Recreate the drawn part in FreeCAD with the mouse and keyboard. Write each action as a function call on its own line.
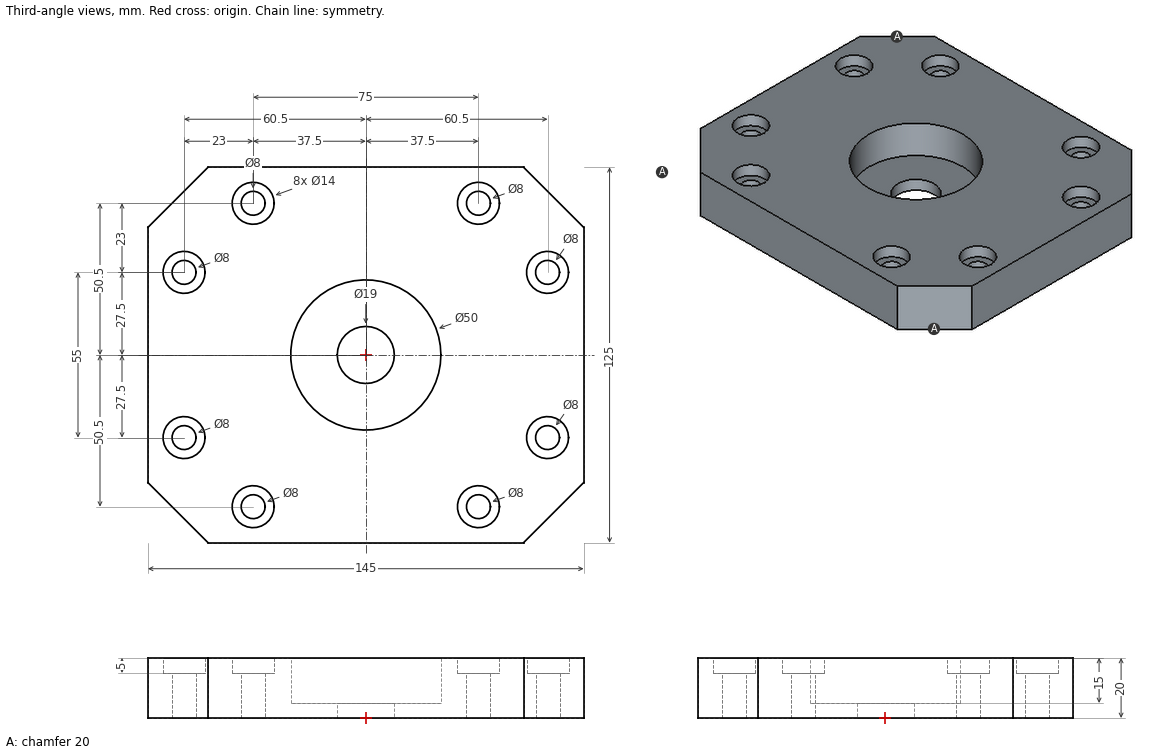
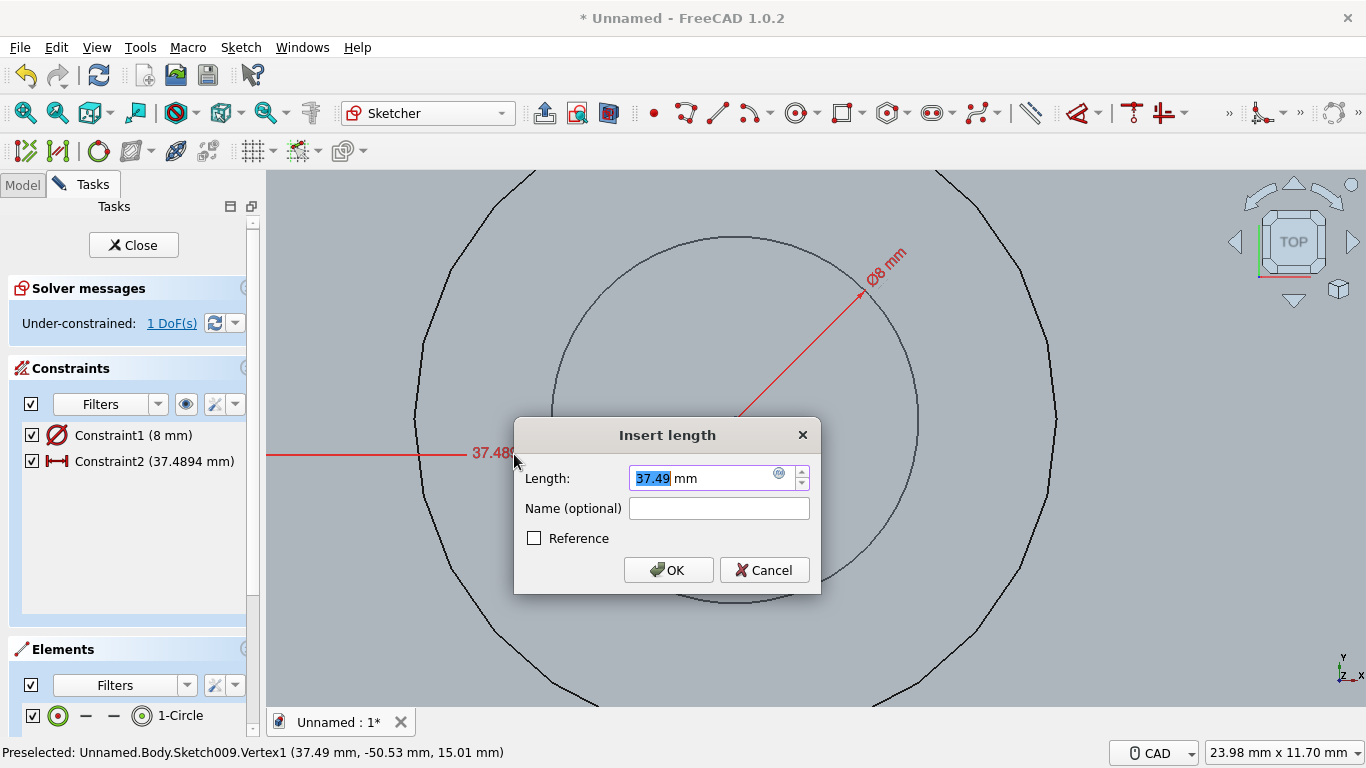
text(37.5)
key(Return)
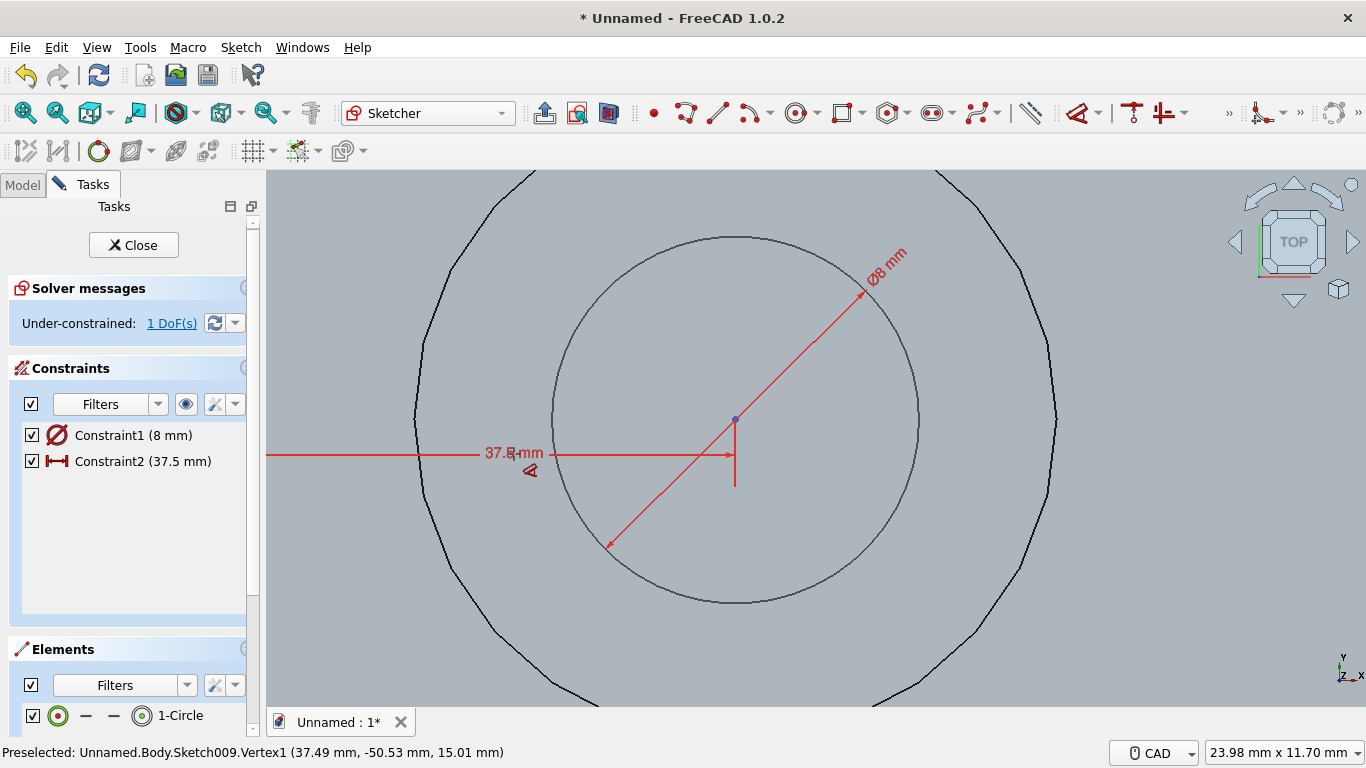
click(735, 420)
click(769, 309)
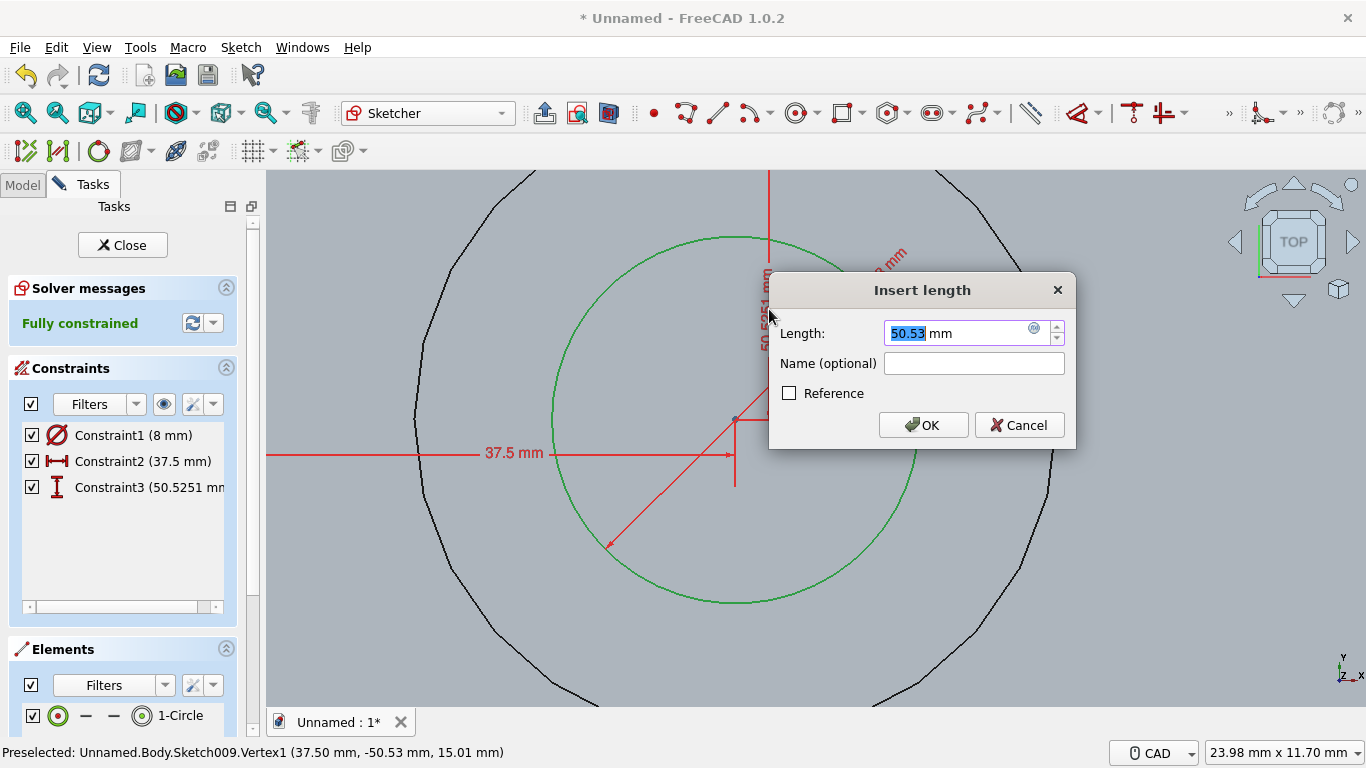
text(50.5)
key(Return)
key(Escape)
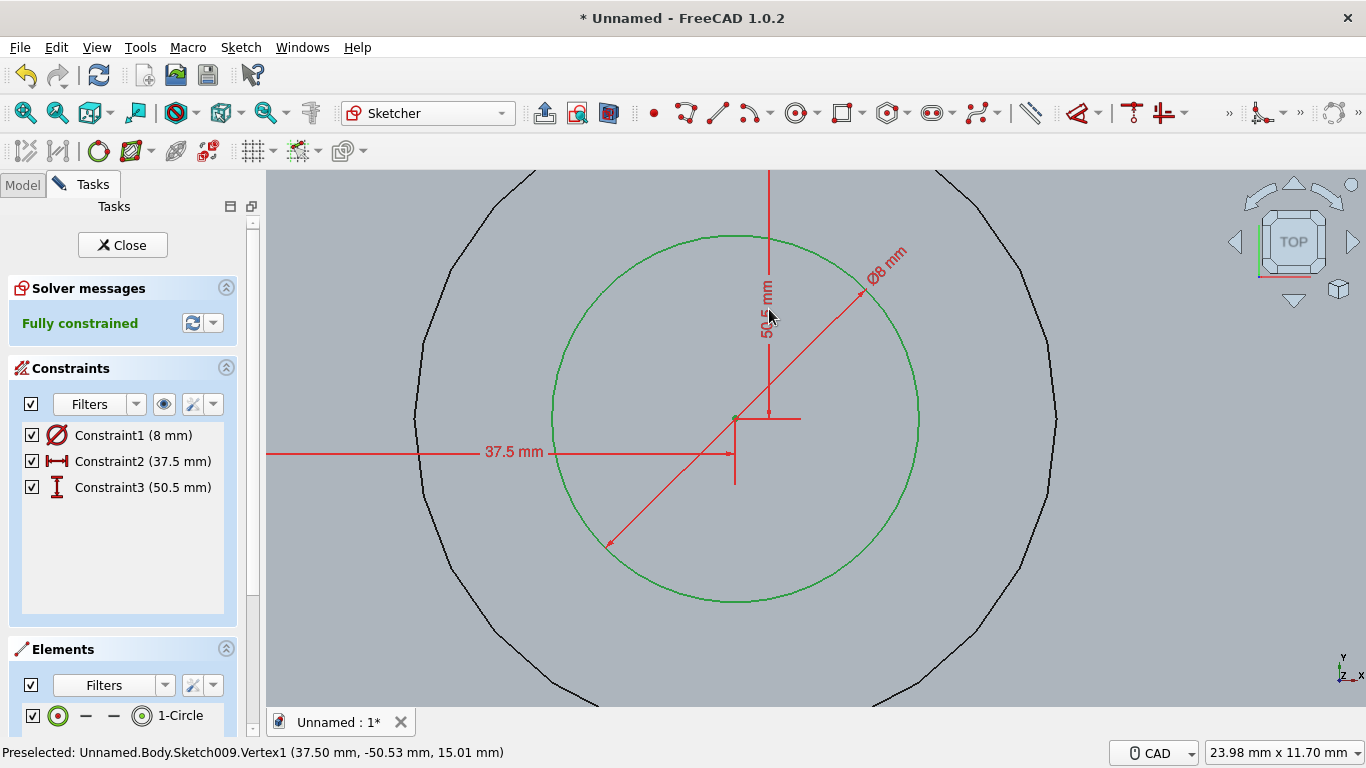
click(123, 245)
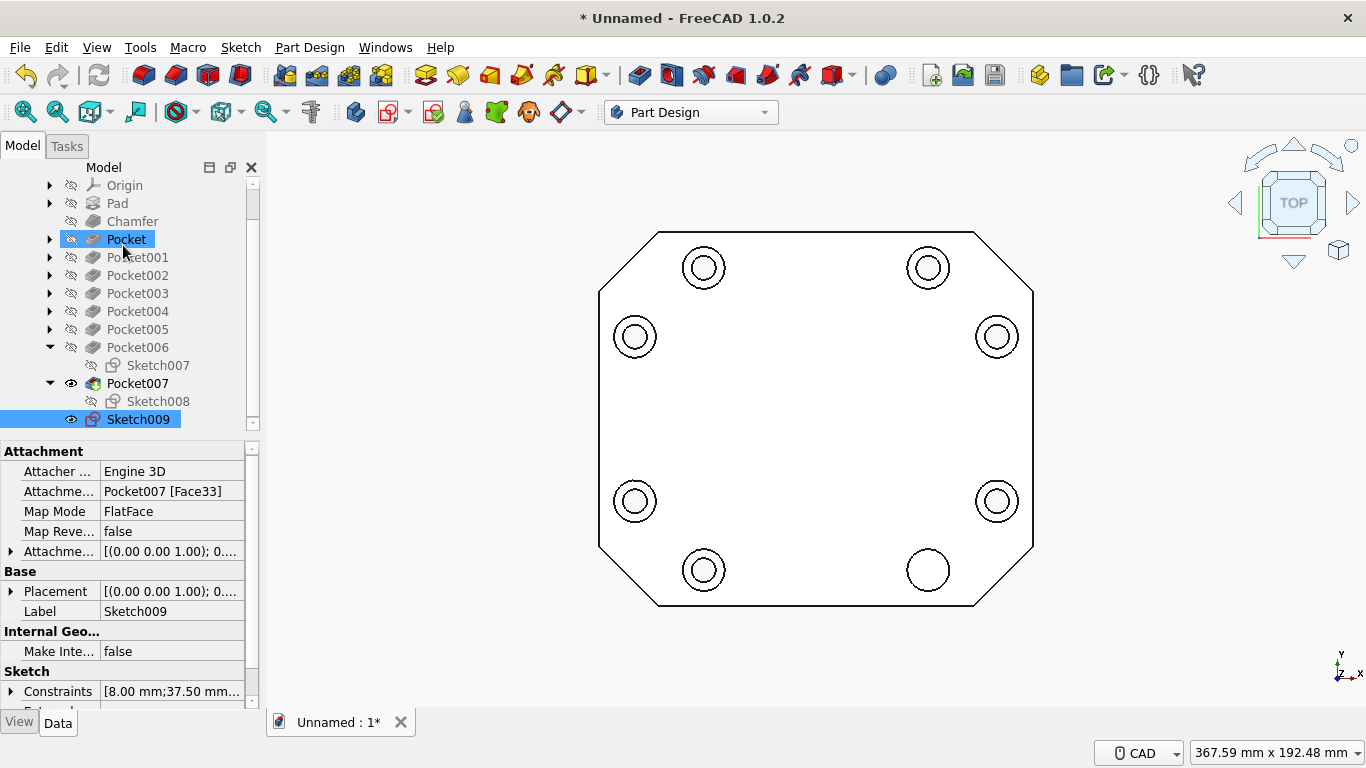
click(640, 76)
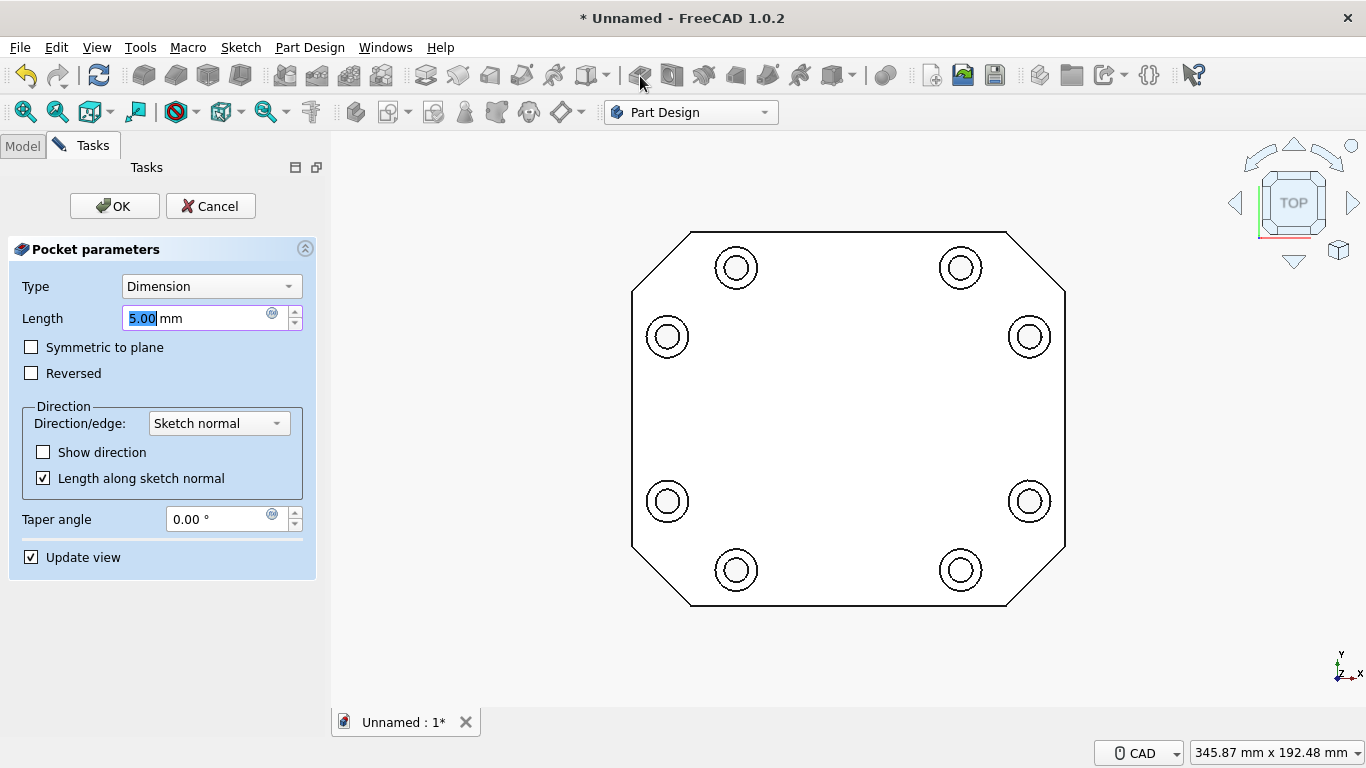
click(212, 286)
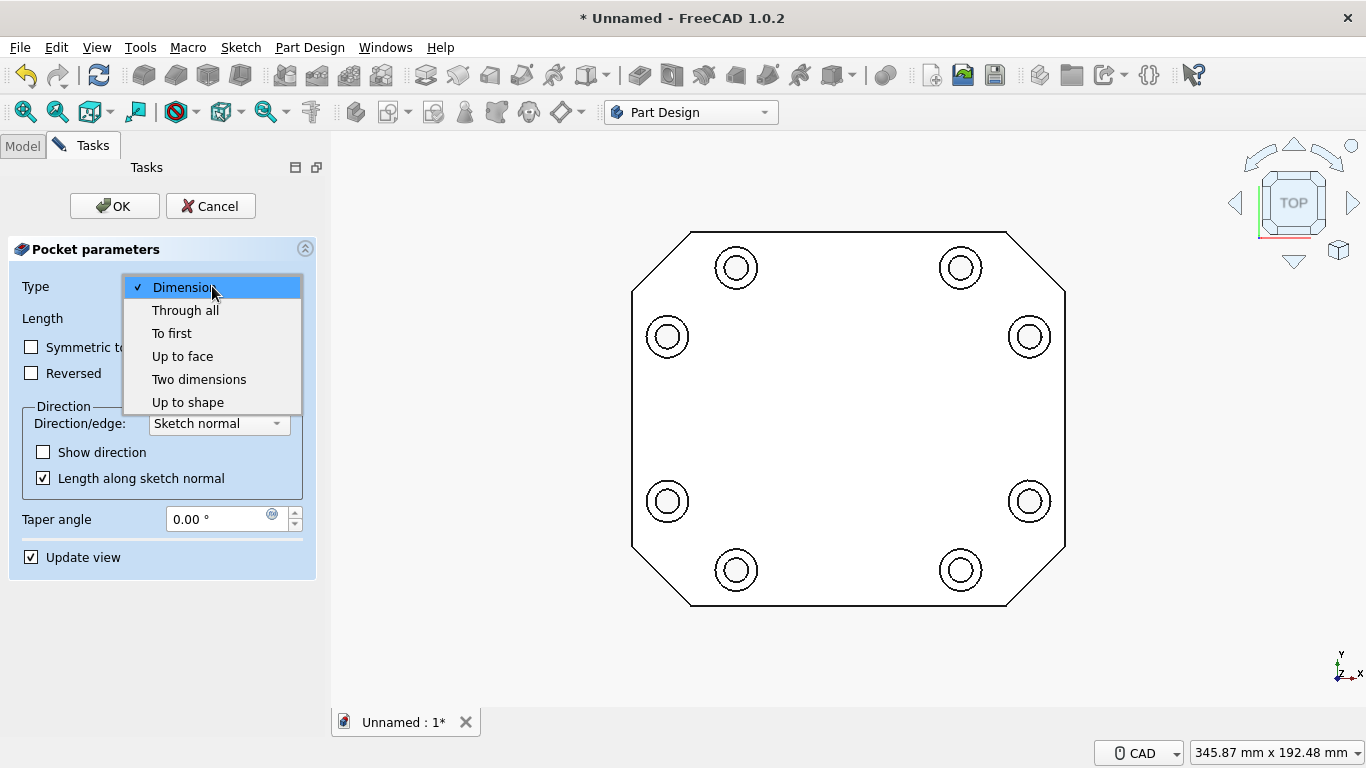
click(212, 334)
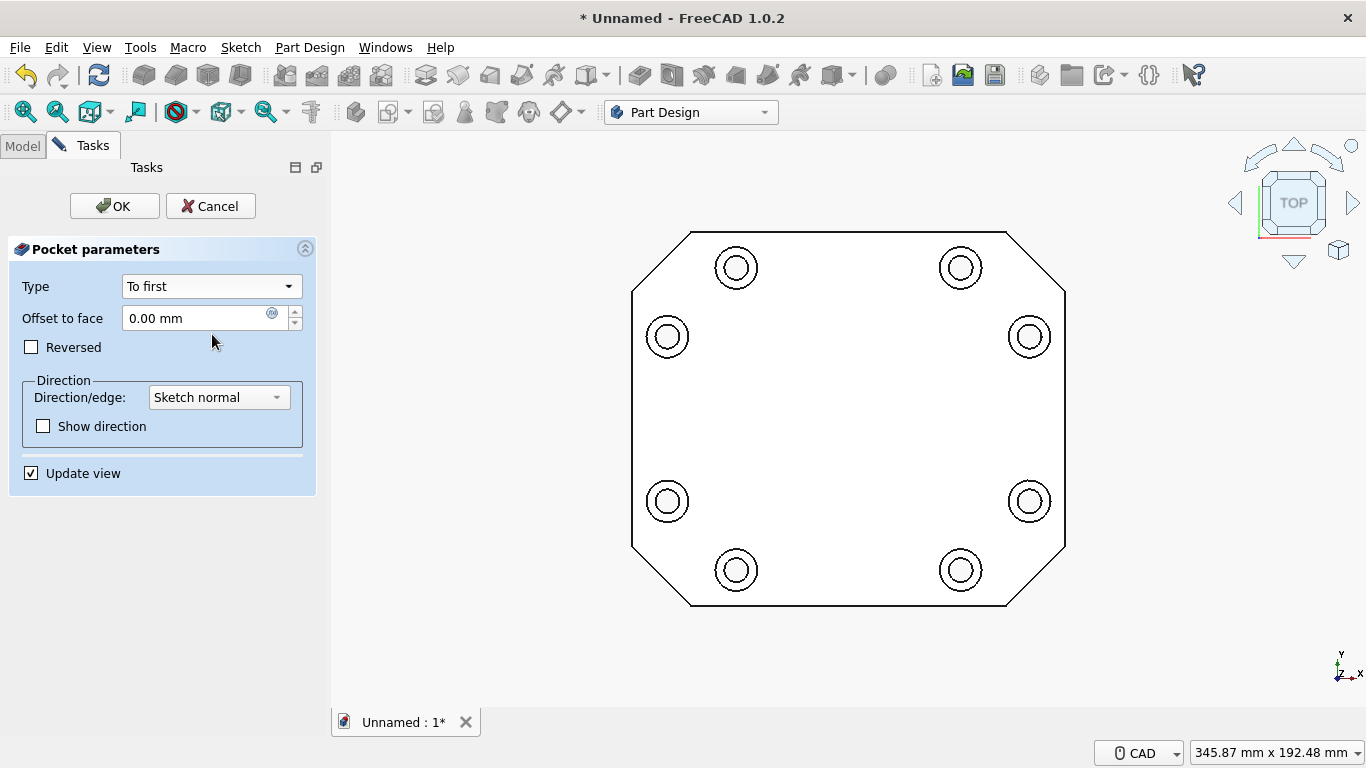
click(115, 206)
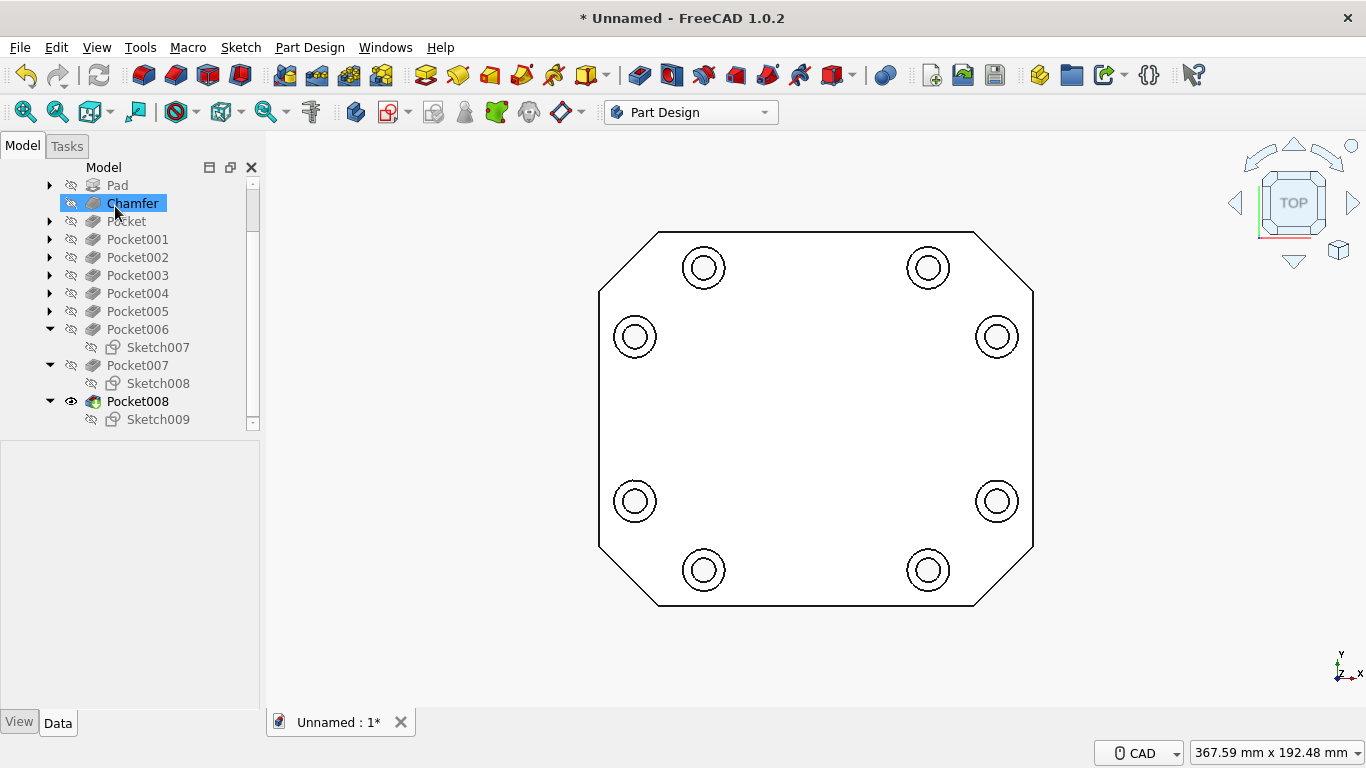
click(388, 112)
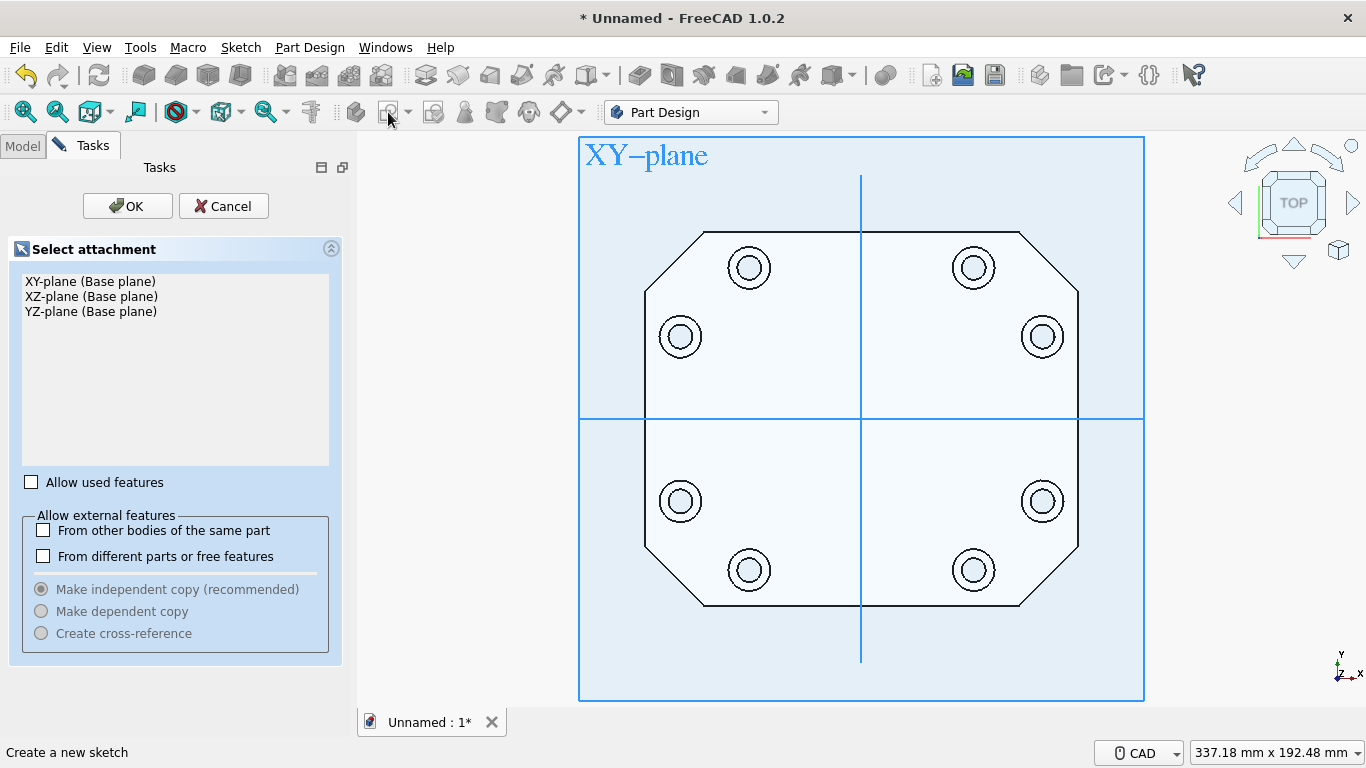
click(82, 282)